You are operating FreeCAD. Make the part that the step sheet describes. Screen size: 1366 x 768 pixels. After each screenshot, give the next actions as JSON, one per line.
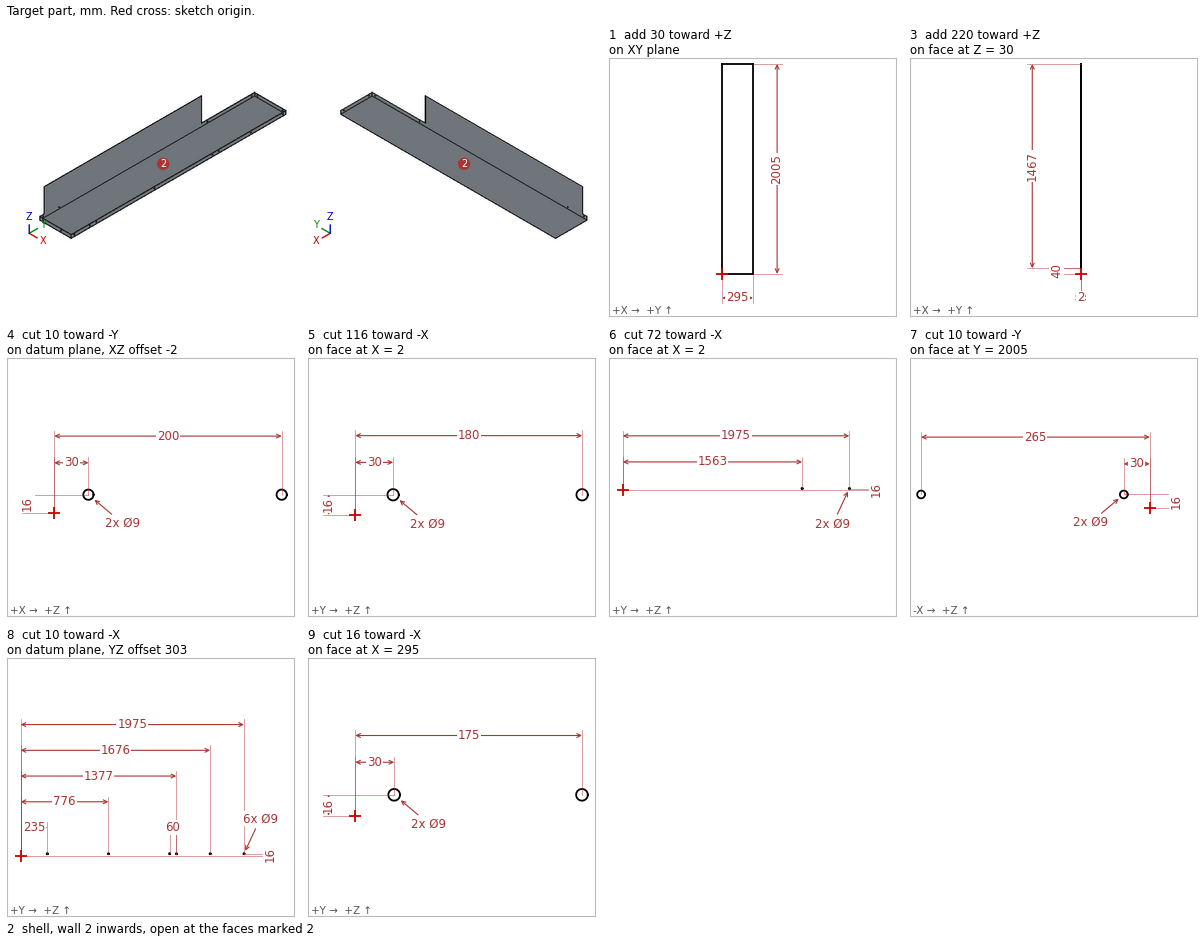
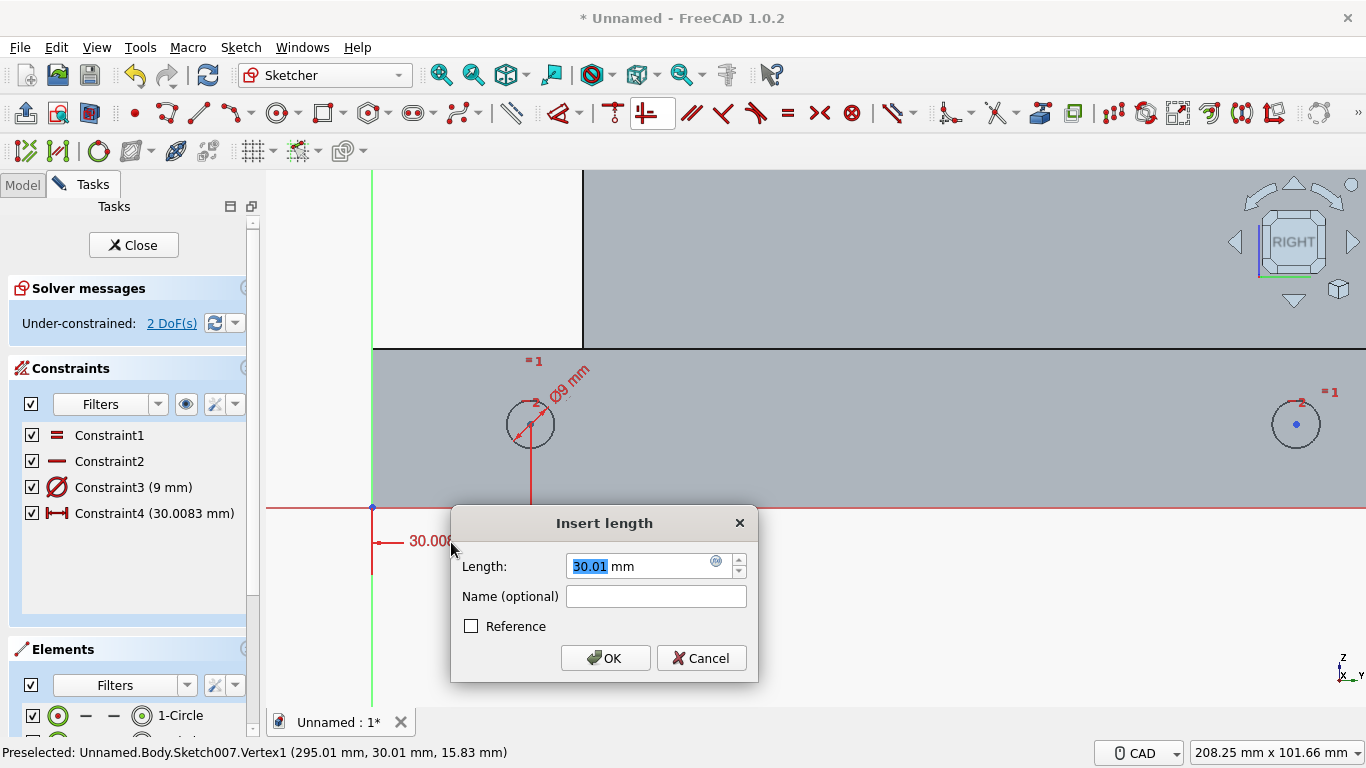
{"action": "type", "text": "30"}
{"action": "key", "text": "Return"}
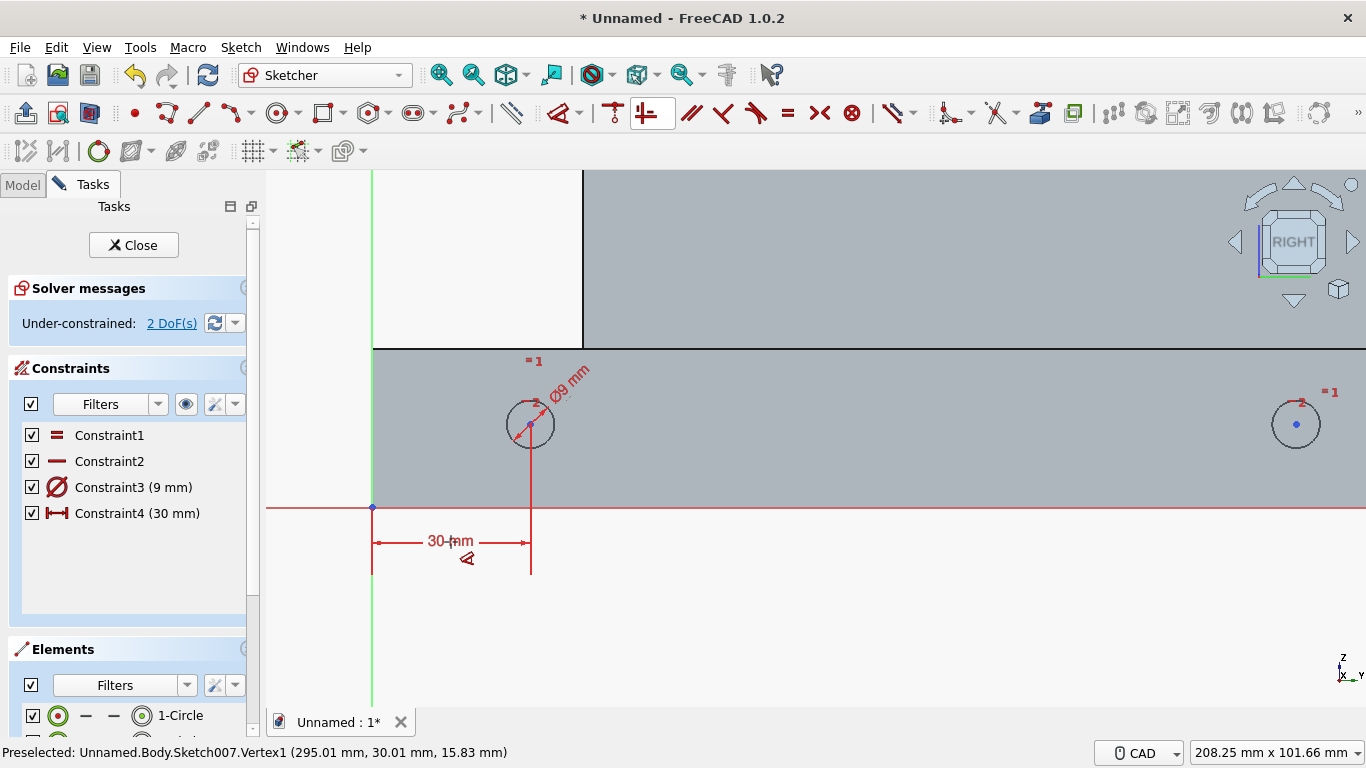
{"action": "left_click", "coordinate": [531, 424]}
{"action": "left_click", "coordinate": [338, 466]}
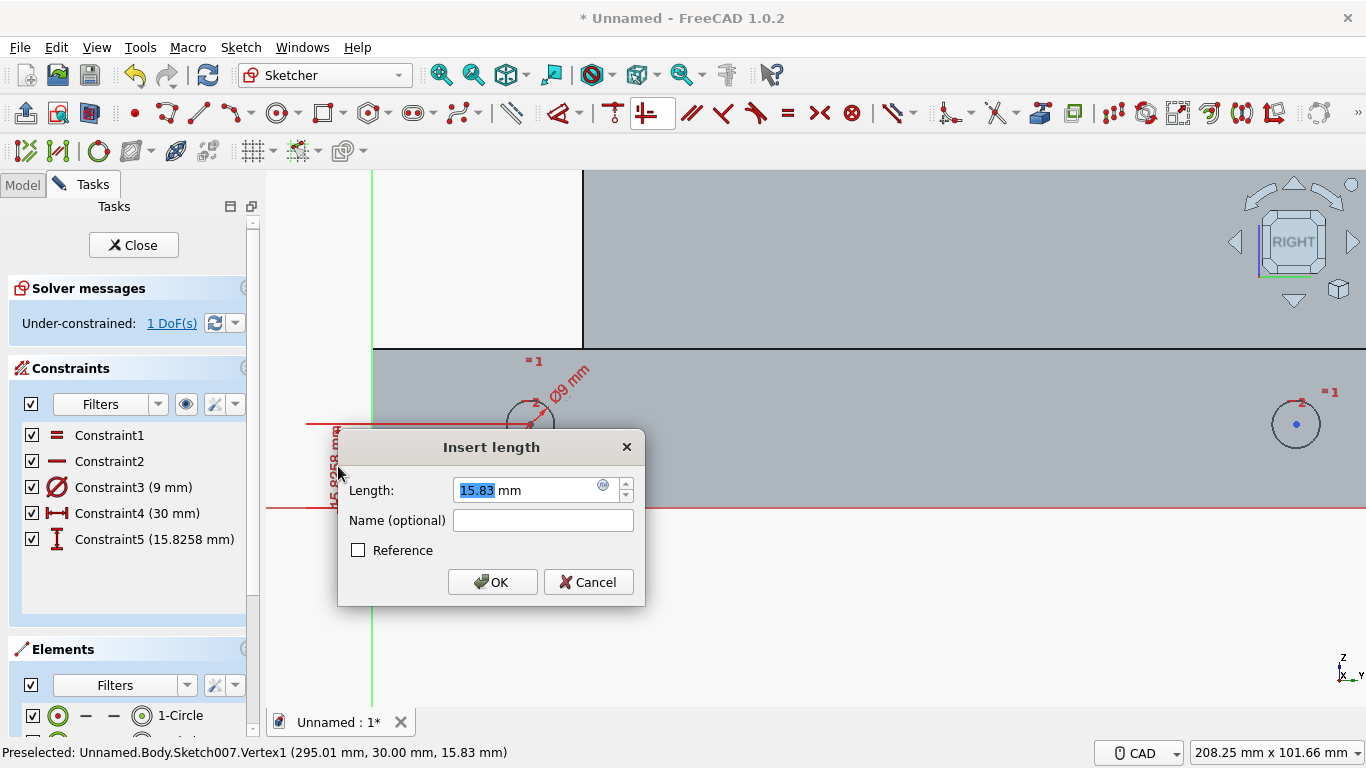
{"action": "type", "text": "16"}
{"action": "key", "text": "Return"}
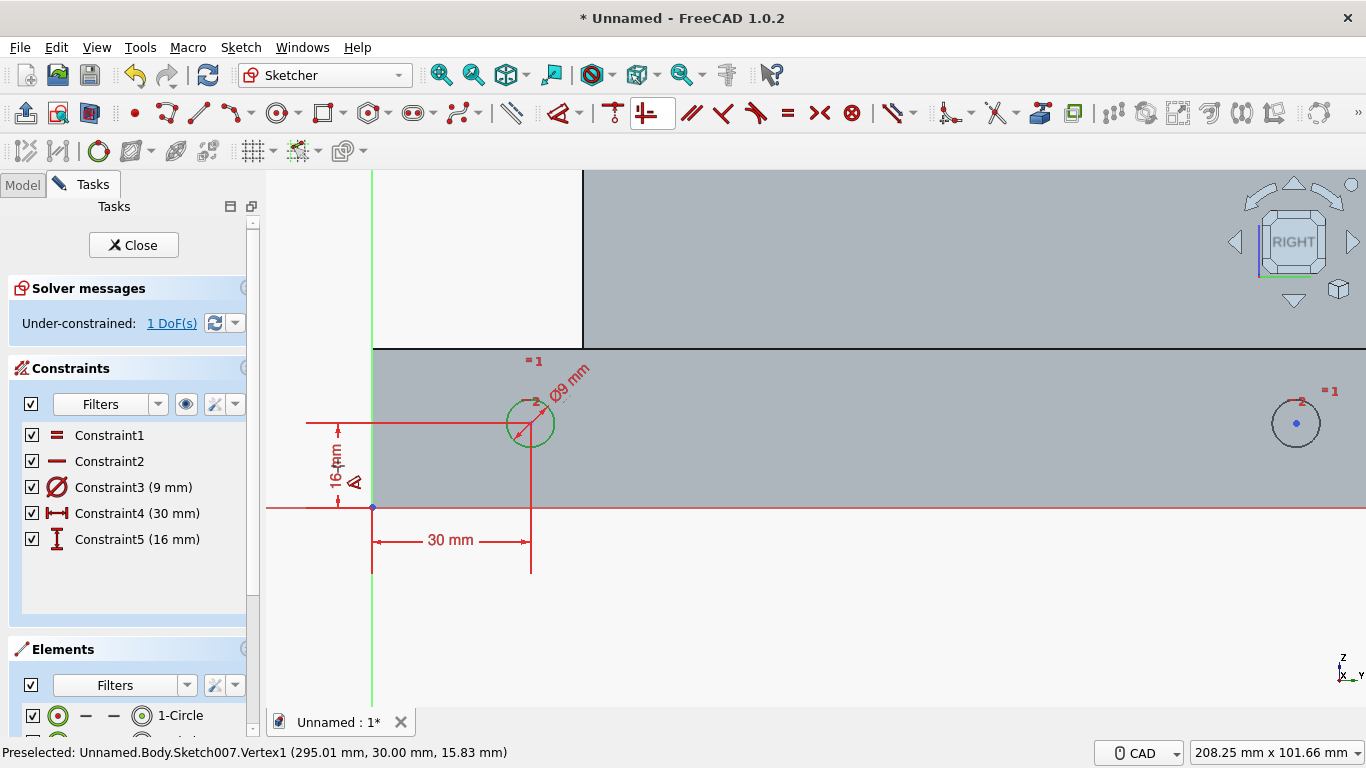
{"action": "scroll", "coordinate": [547, 407], "scroll_direction": "down", "scroll_amount": 2}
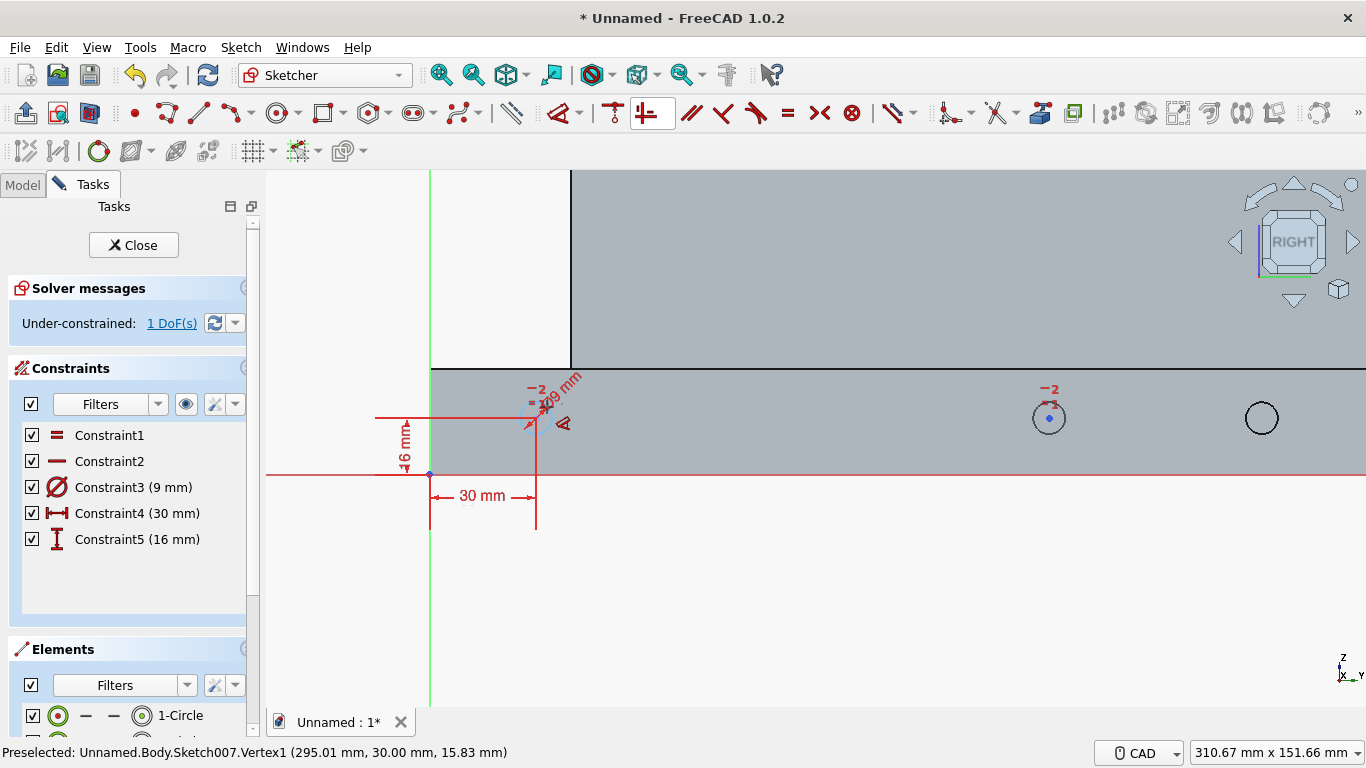
{"action": "left_click", "coordinate": [1049, 418]}
{"action": "left_click", "coordinate": [740, 509]}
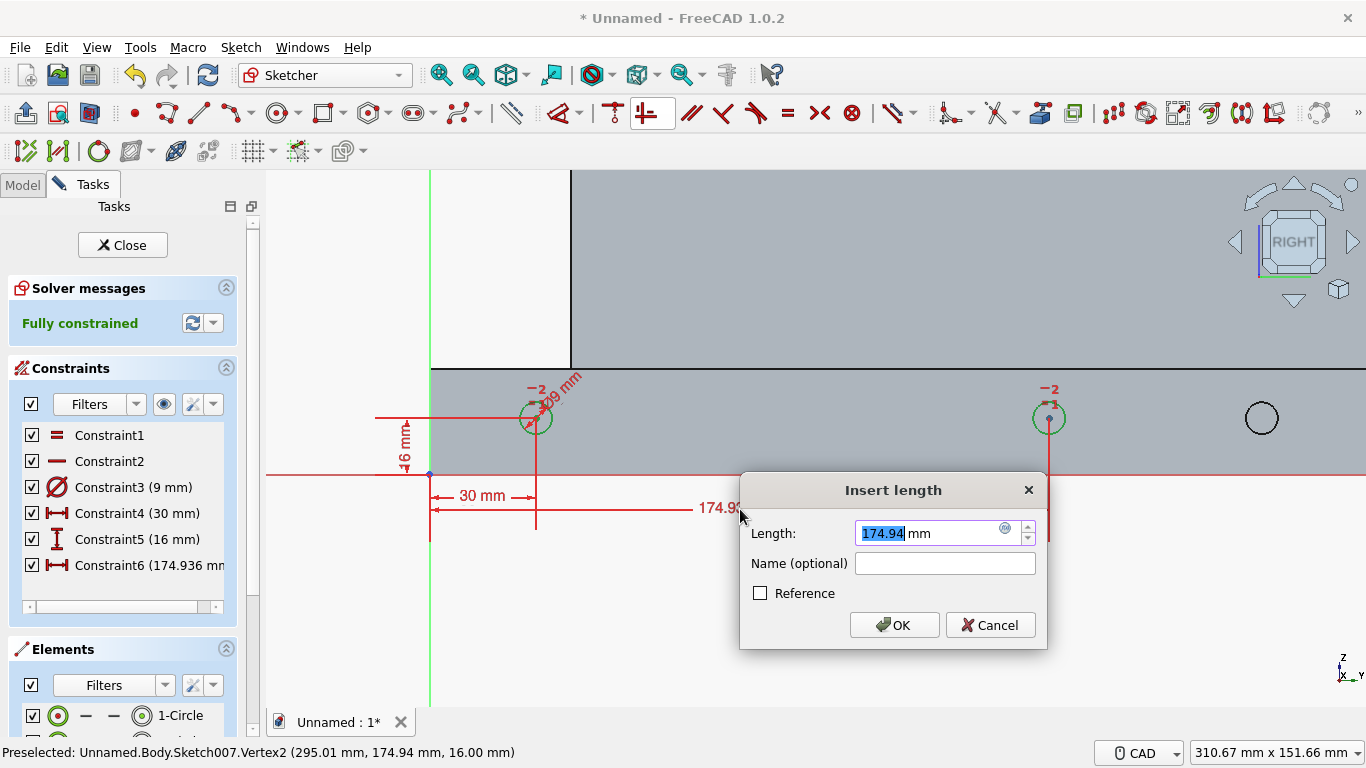
{"action": "type", "text": "175"}
{"action": "key", "text": "Return"}
{"action": "key", "text": "Escape"}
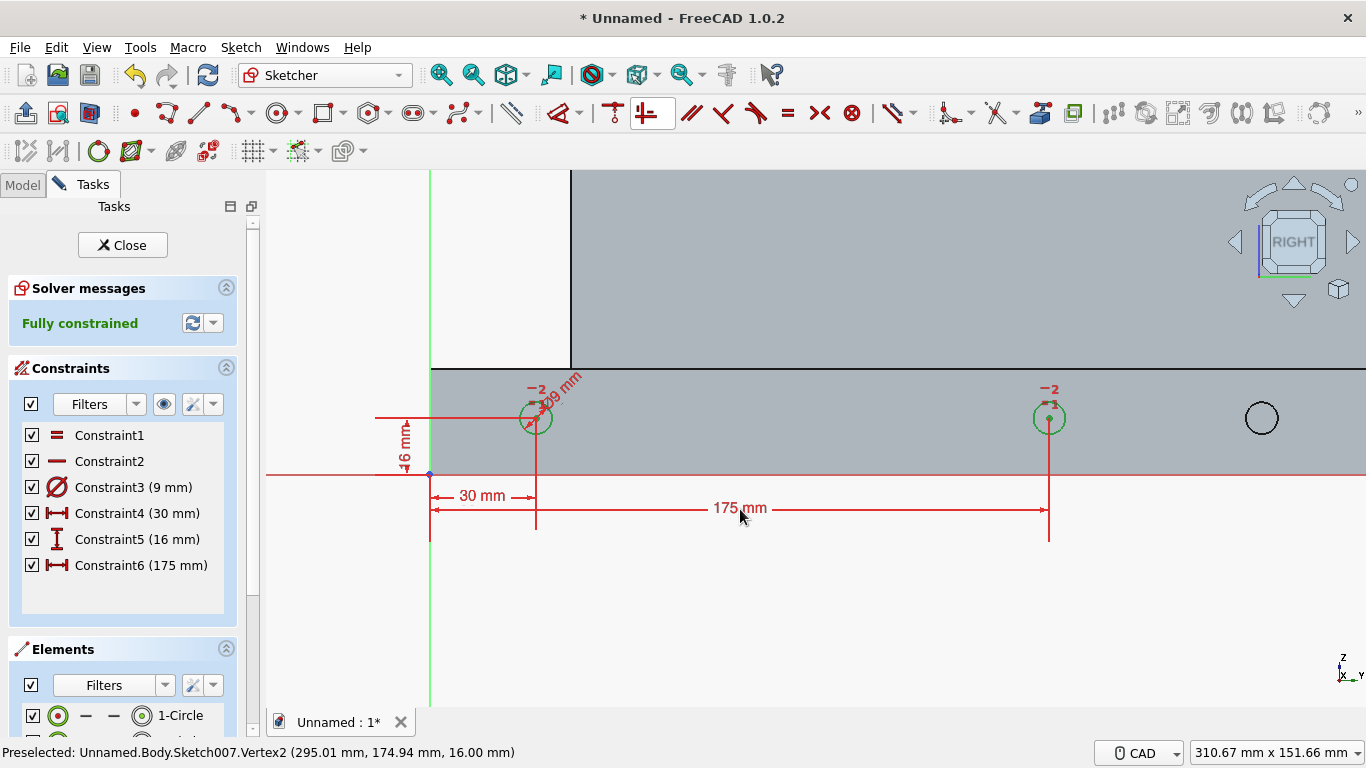
{"action": "left_click", "coordinate": [123, 245]}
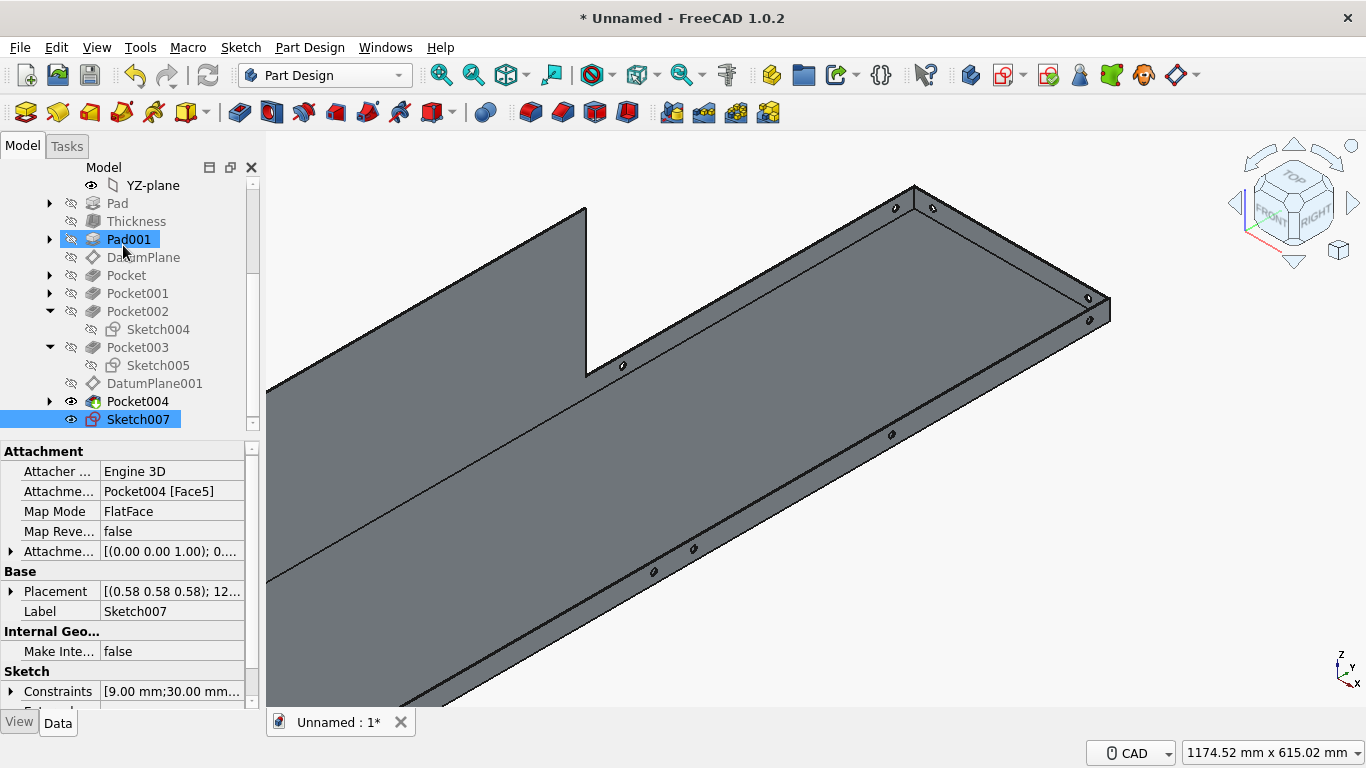
{"action": "left_click", "coordinate": [240, 112]}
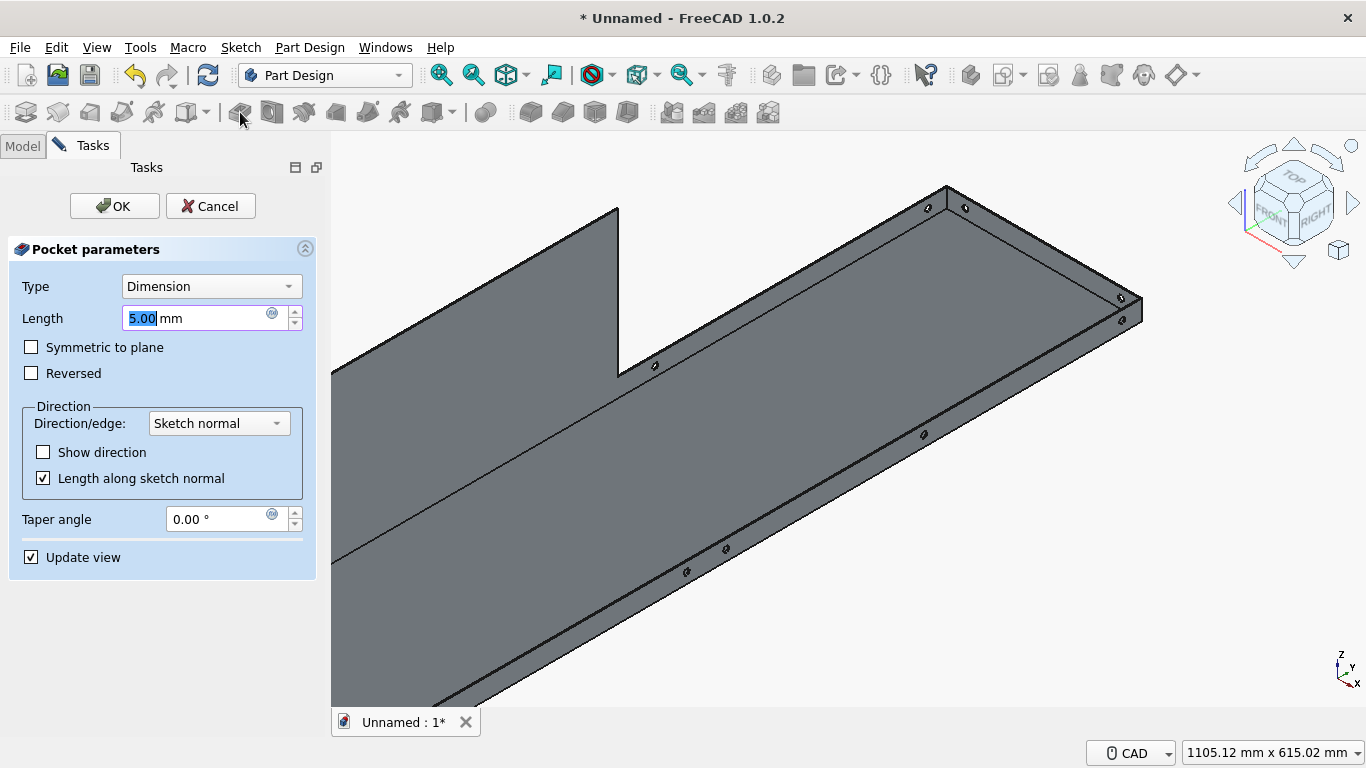
{"action": "type", "text": "16"}
{"action": "key", "text": "Tab"}